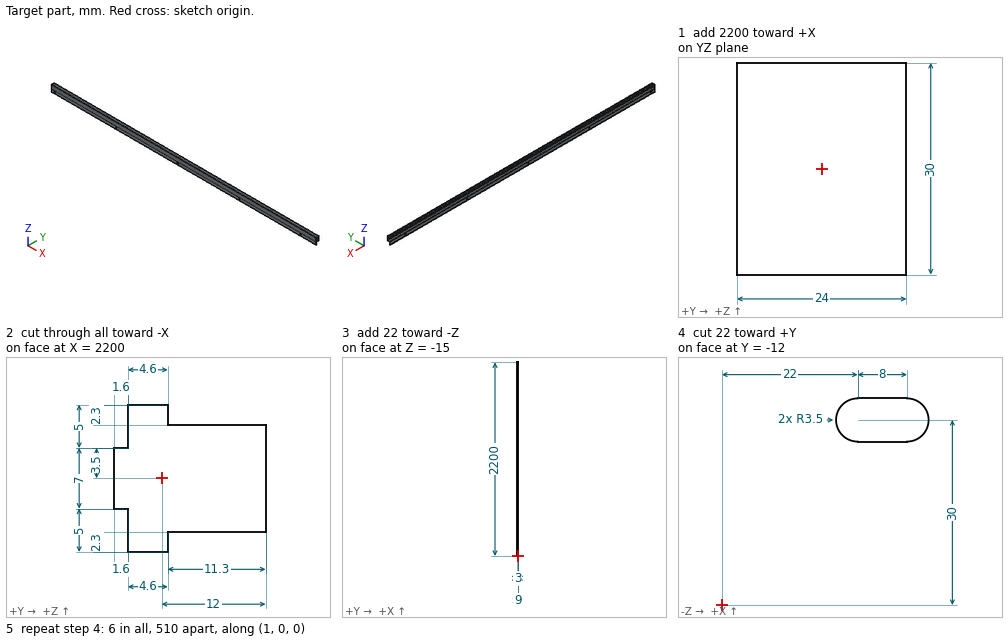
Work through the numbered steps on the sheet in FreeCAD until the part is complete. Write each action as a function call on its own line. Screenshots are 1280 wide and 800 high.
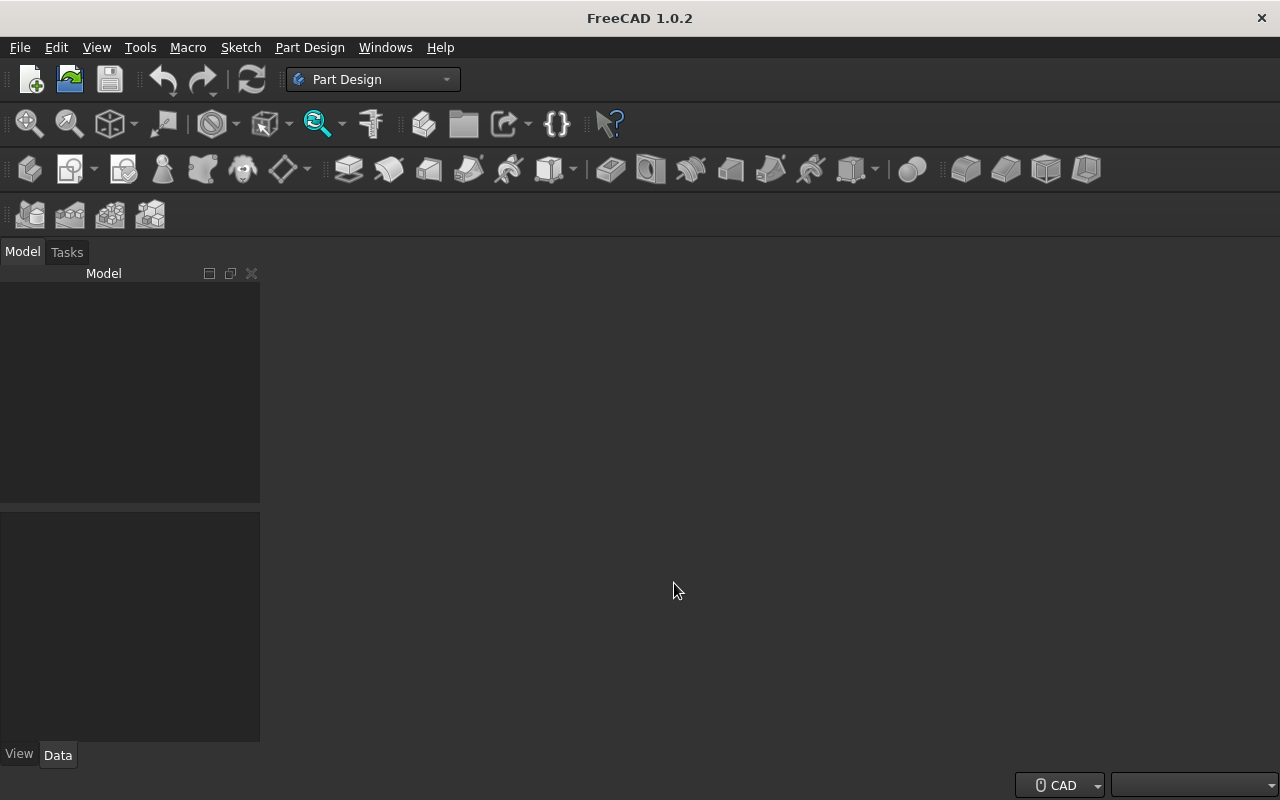
click(30, 80)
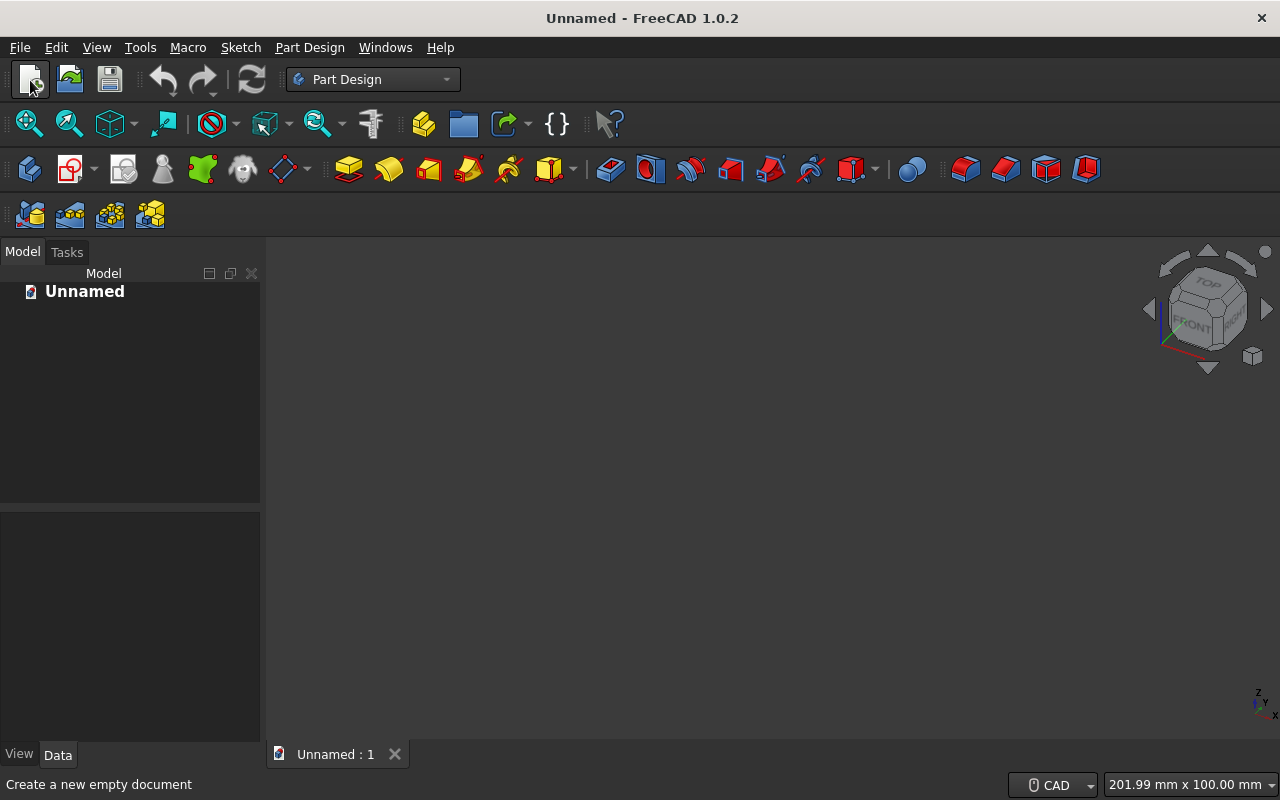
click(70, 170)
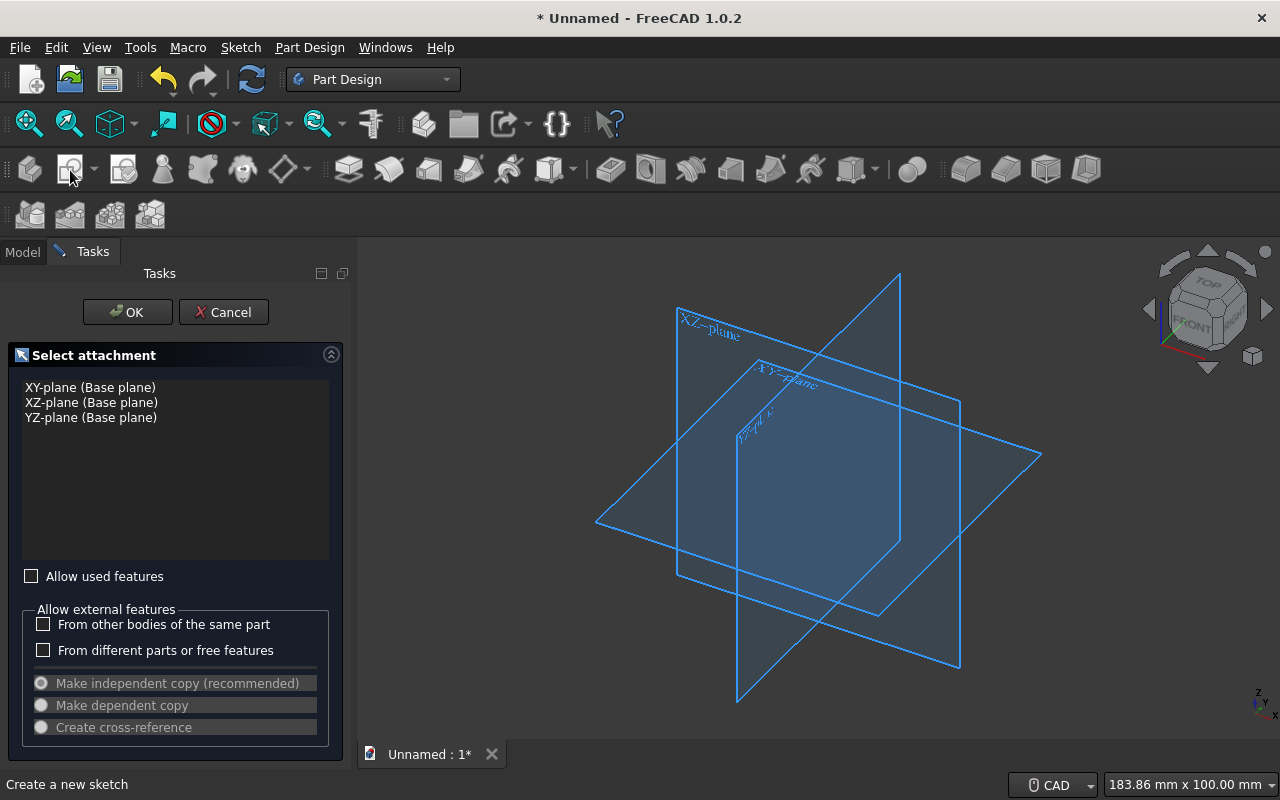
click(82, 418)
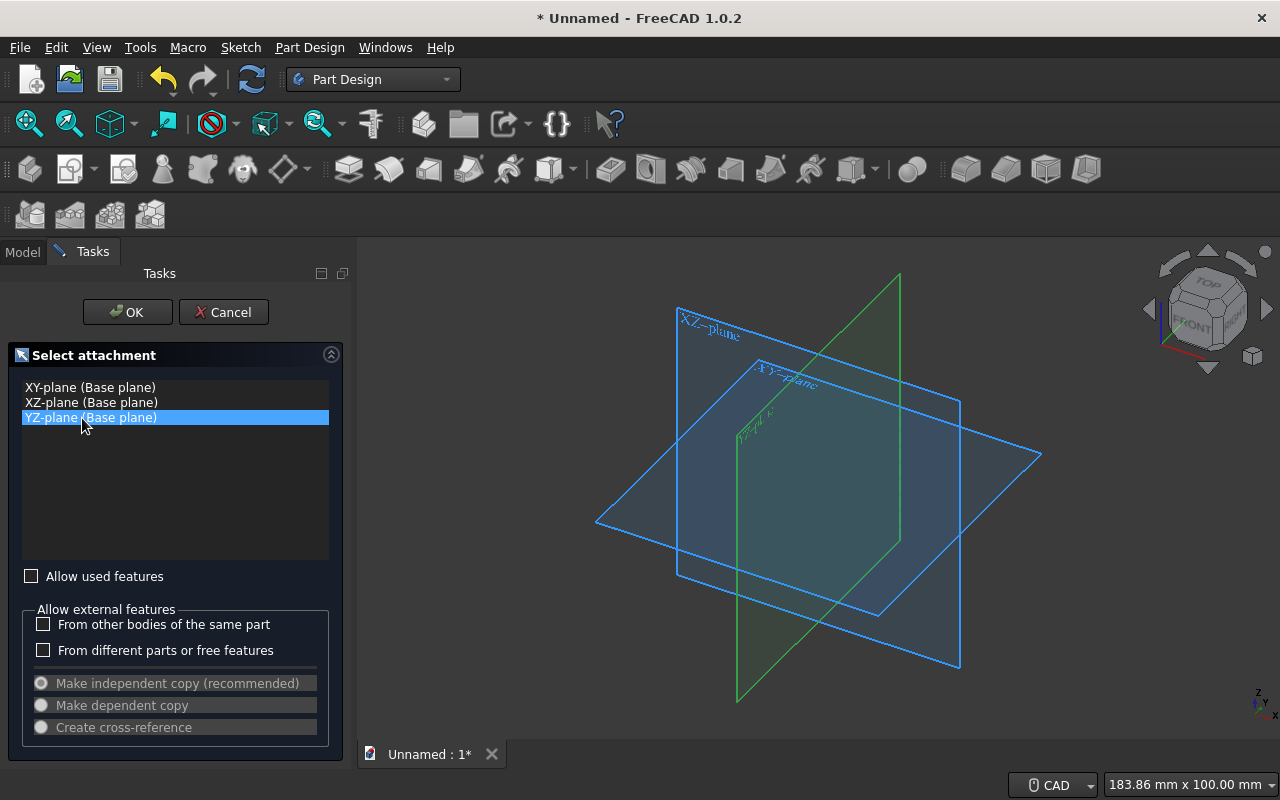
click(128, 312)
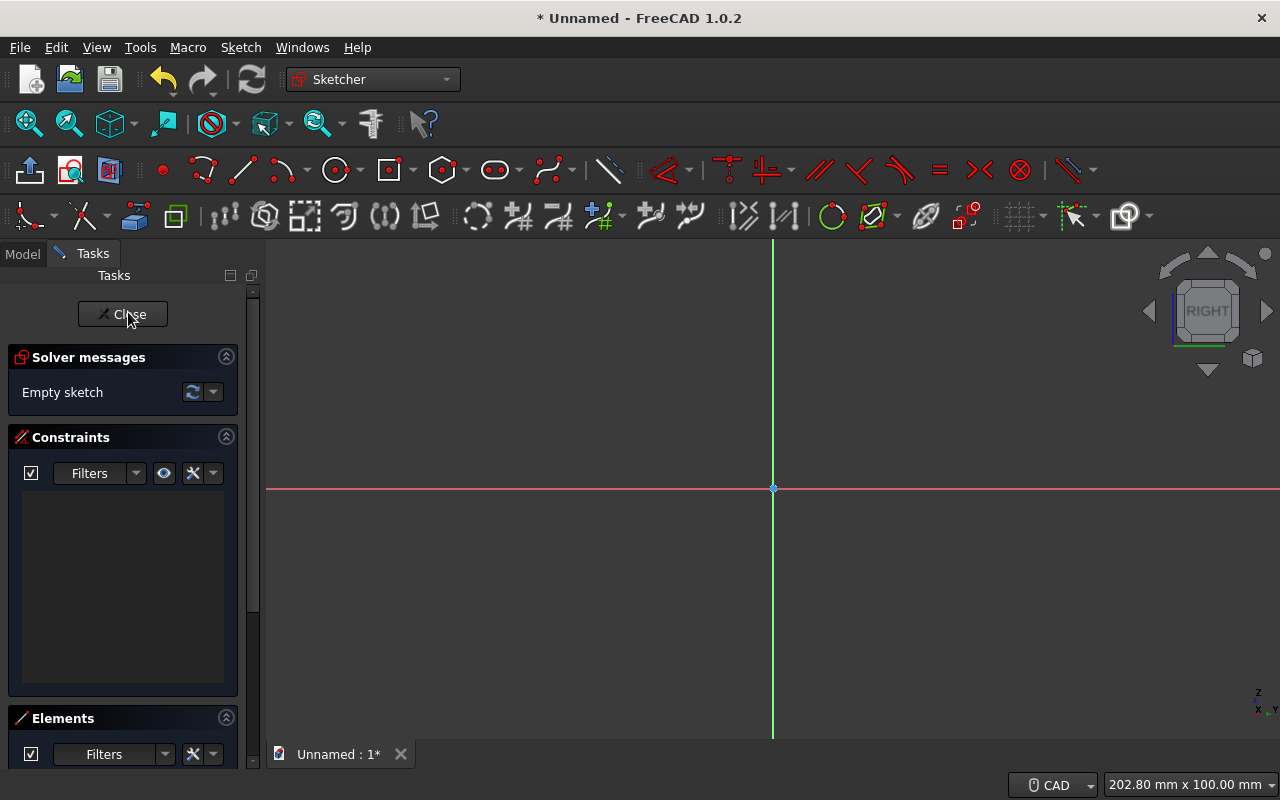
scroll(829, 489, up, 4)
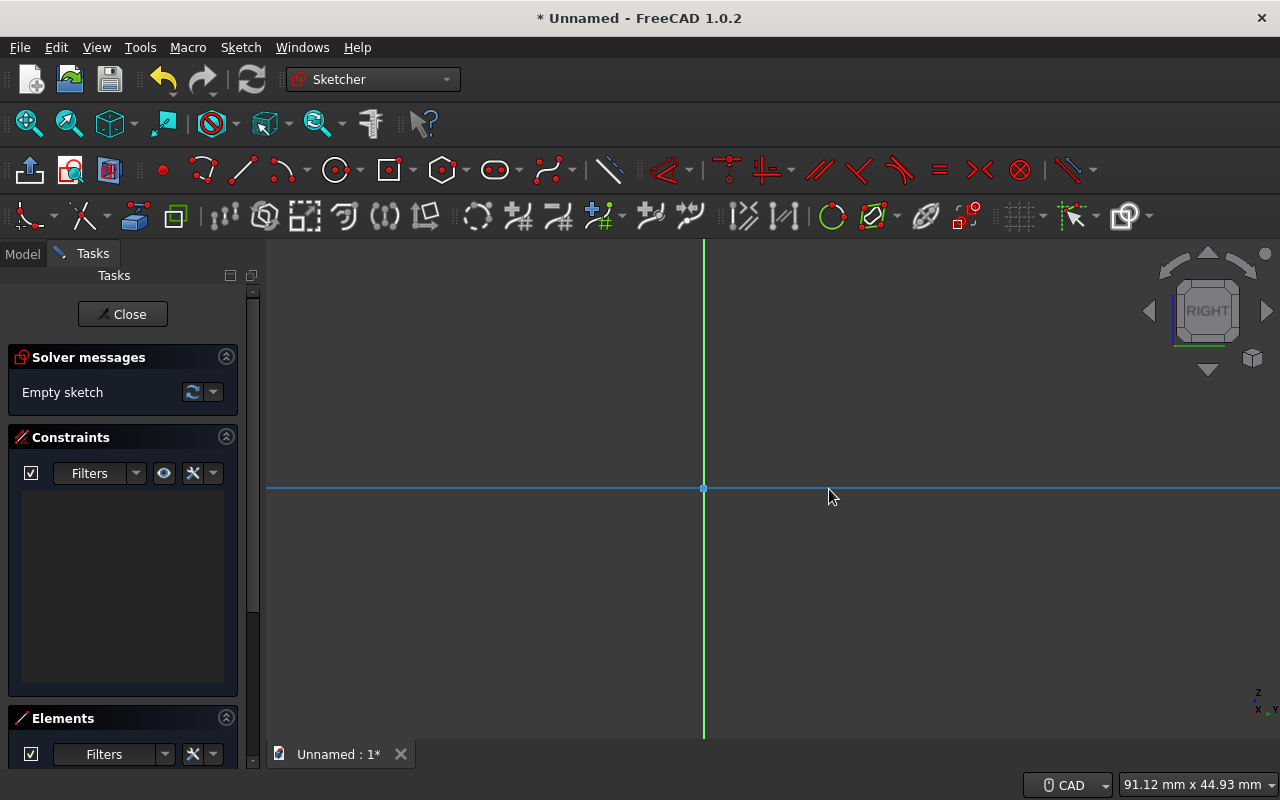
click(390, 170)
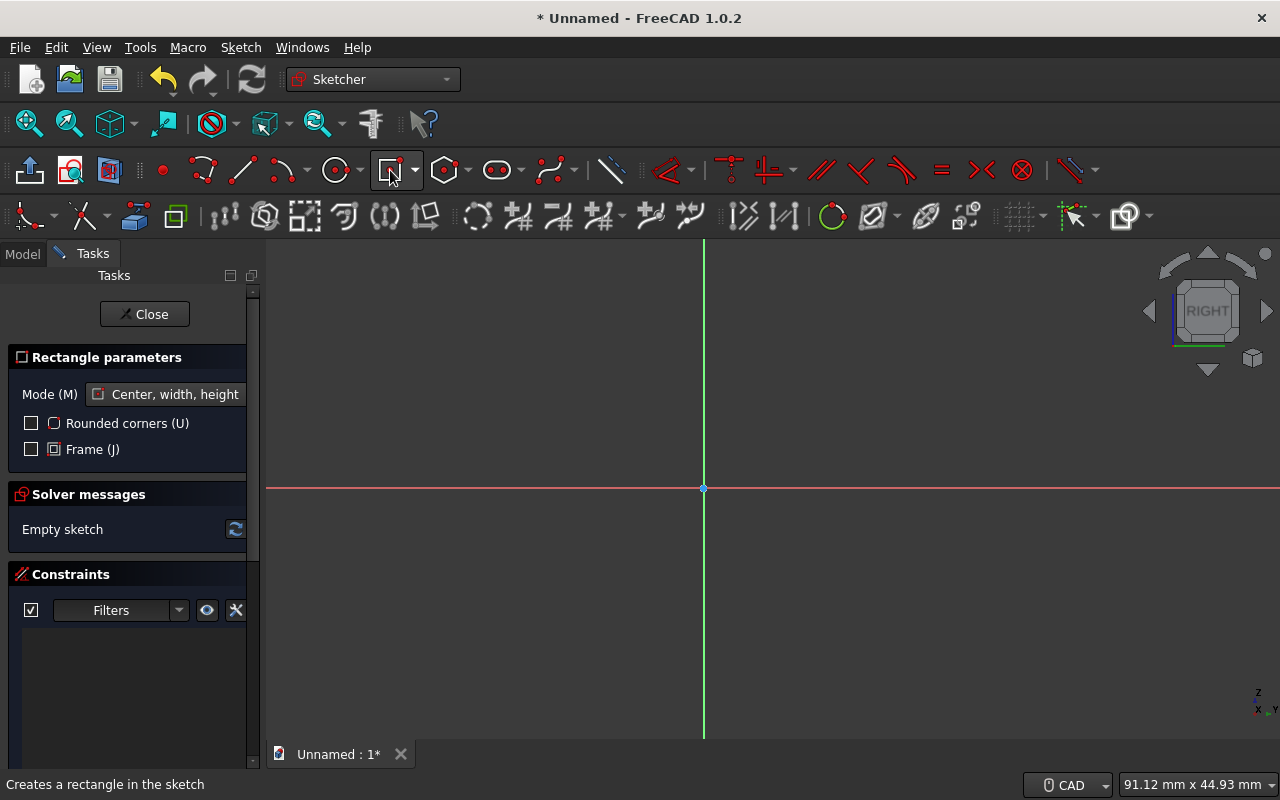
click(704, 488)
click(837, 321)
key(Escape)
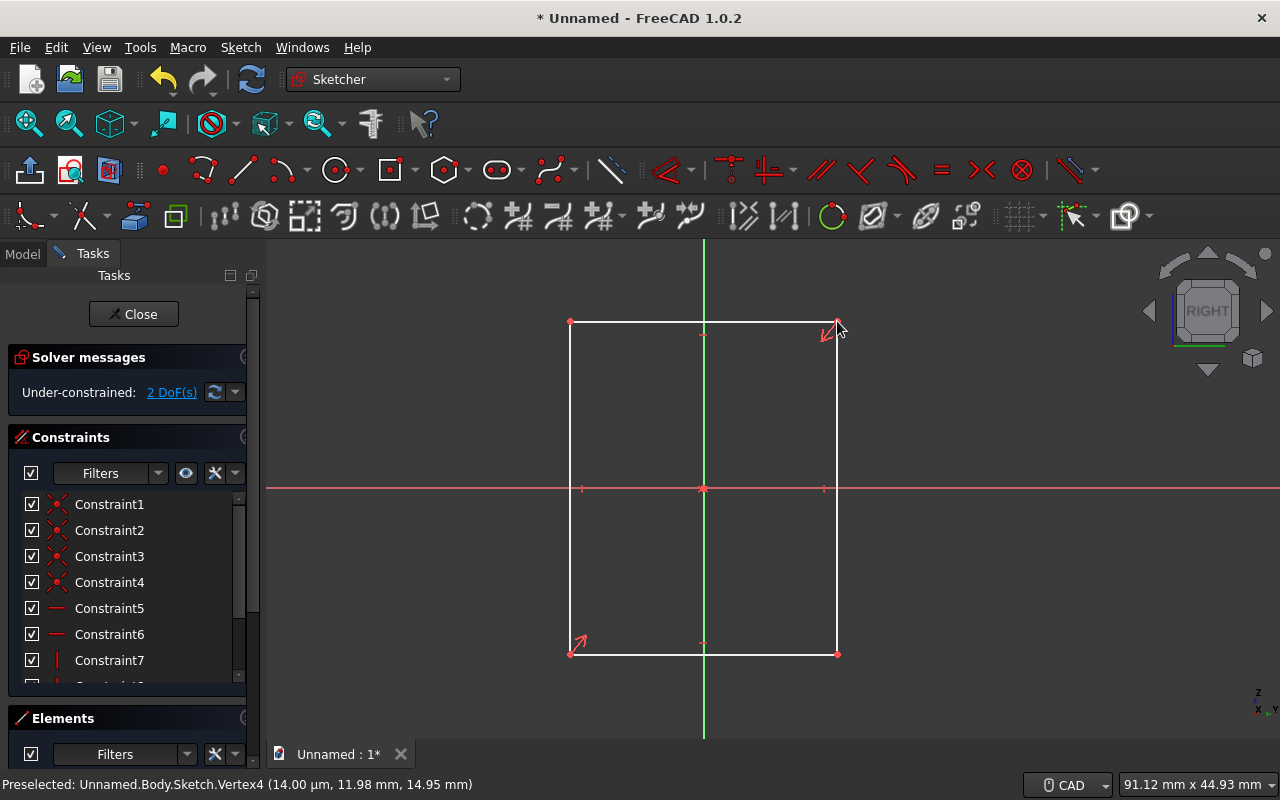
click(650, 655)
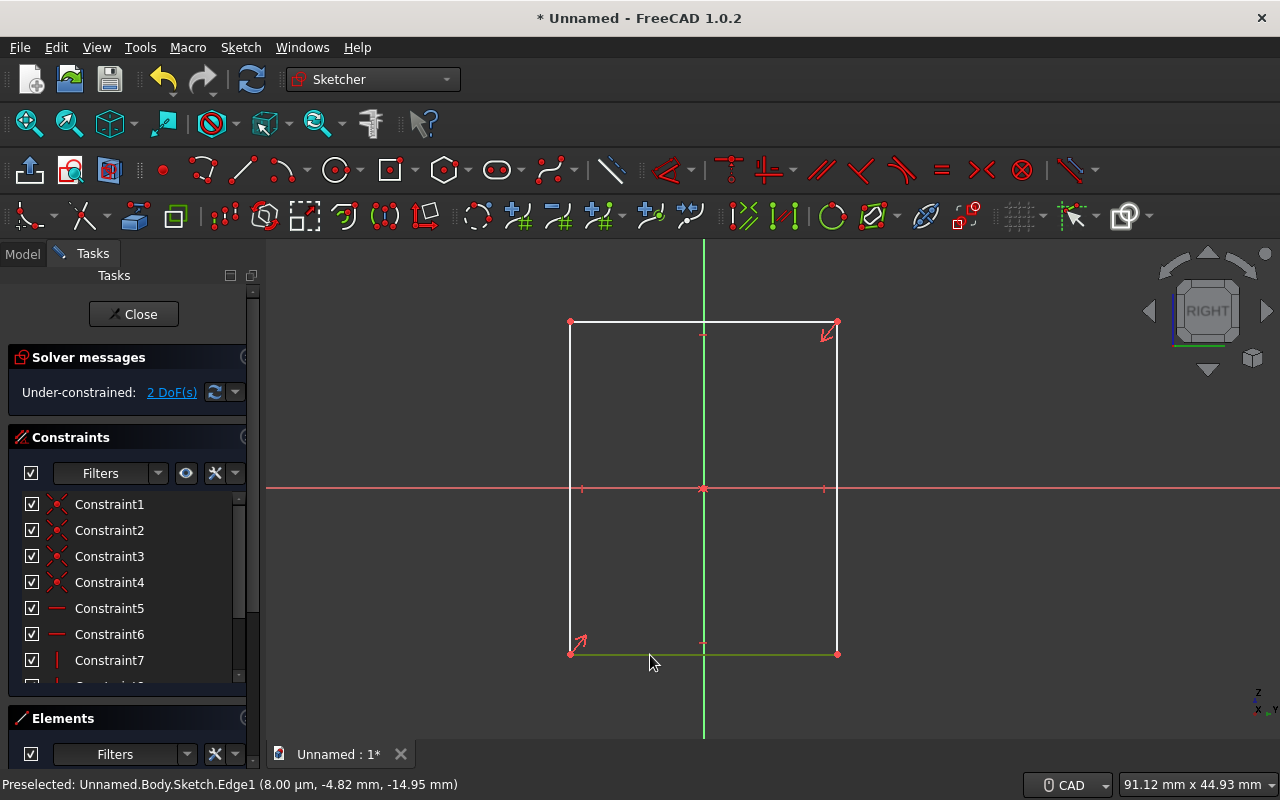
key(l)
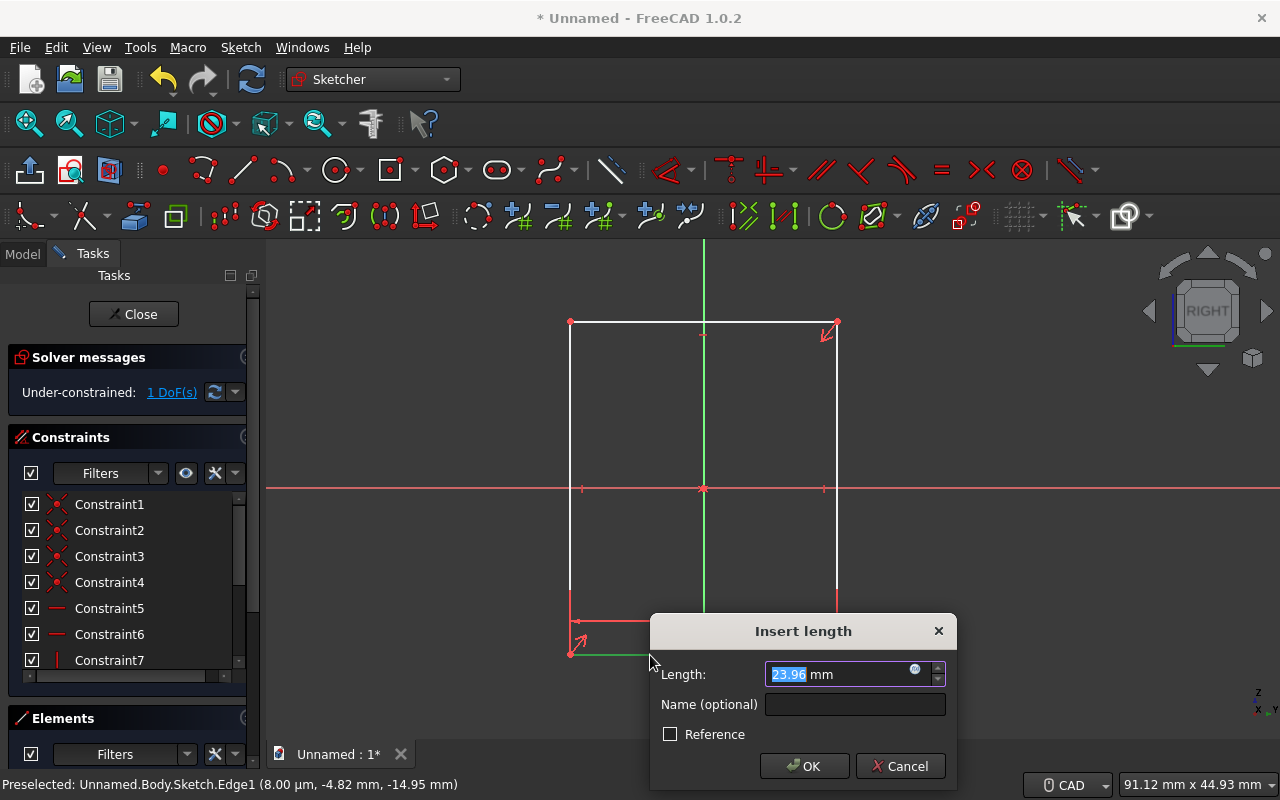
text(24)
key(Return)